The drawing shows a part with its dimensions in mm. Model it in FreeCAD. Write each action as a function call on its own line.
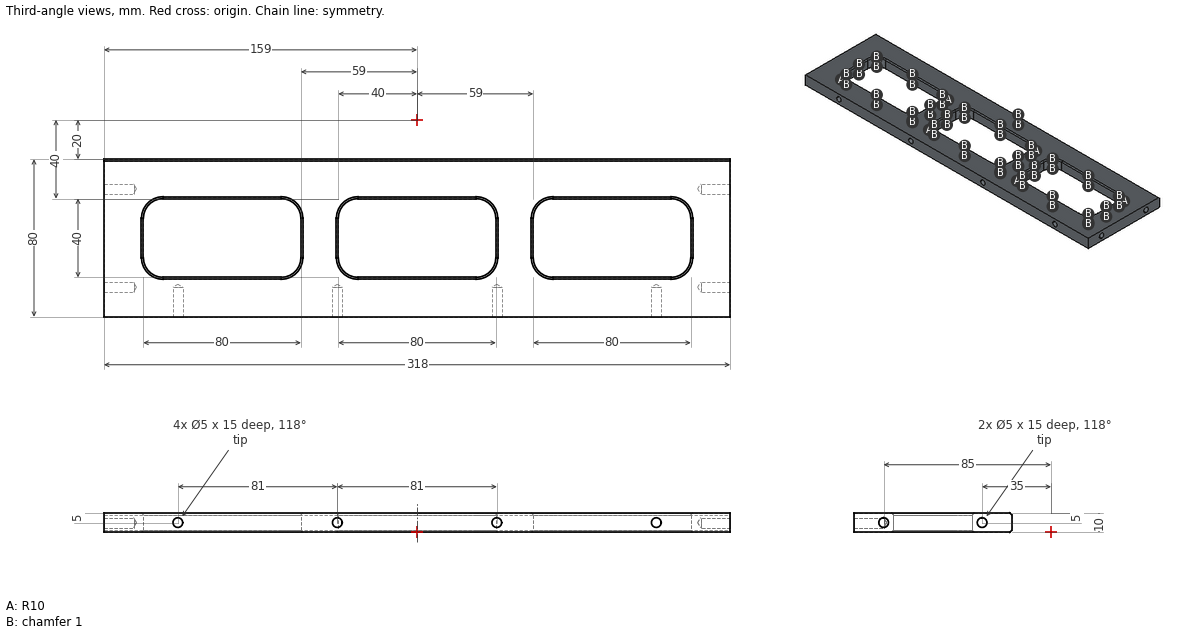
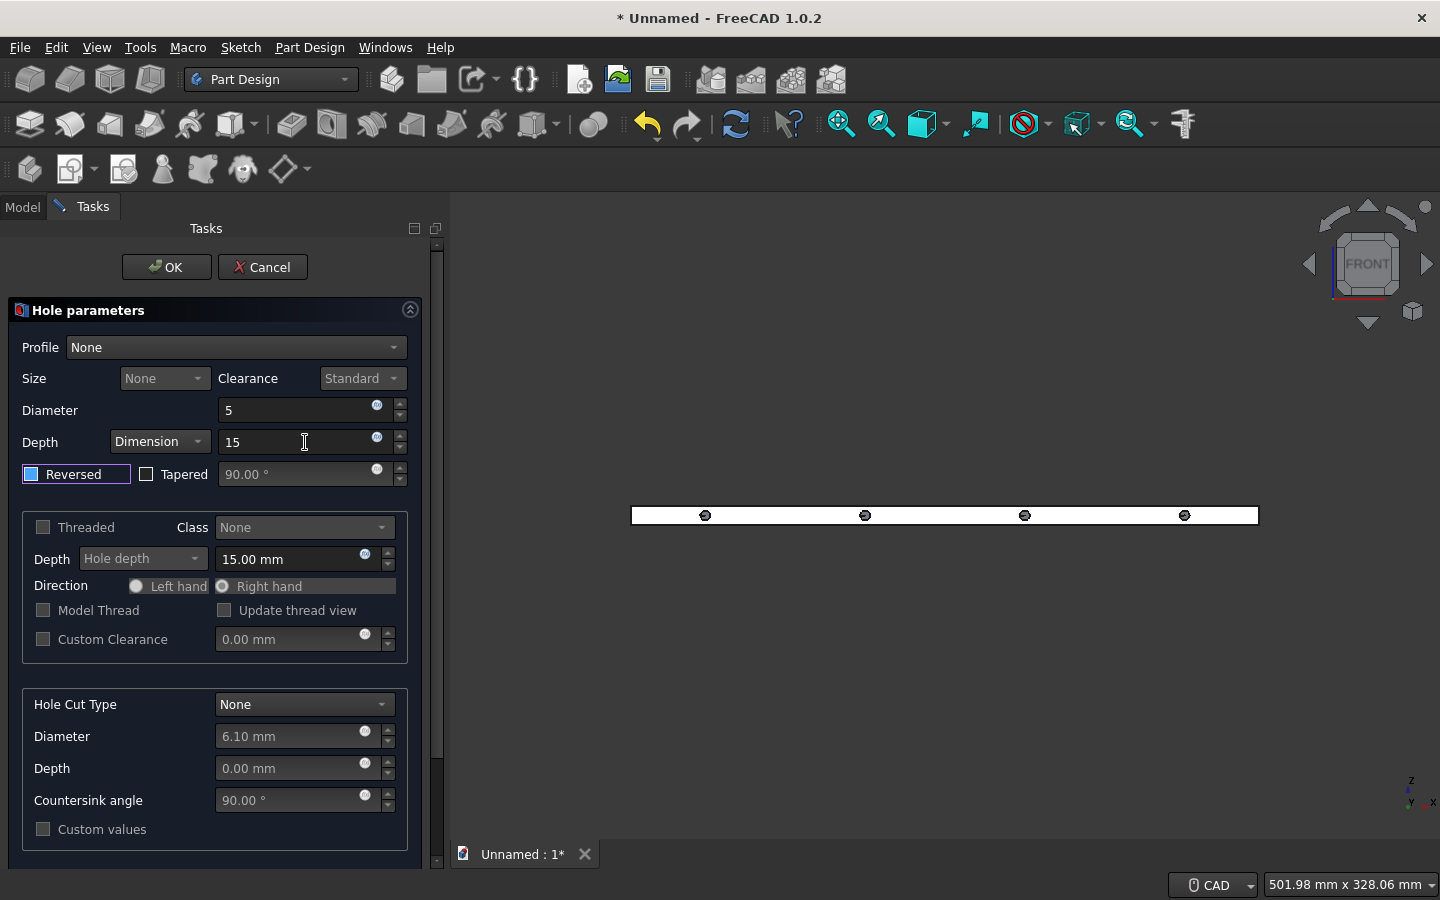
click(167, 267)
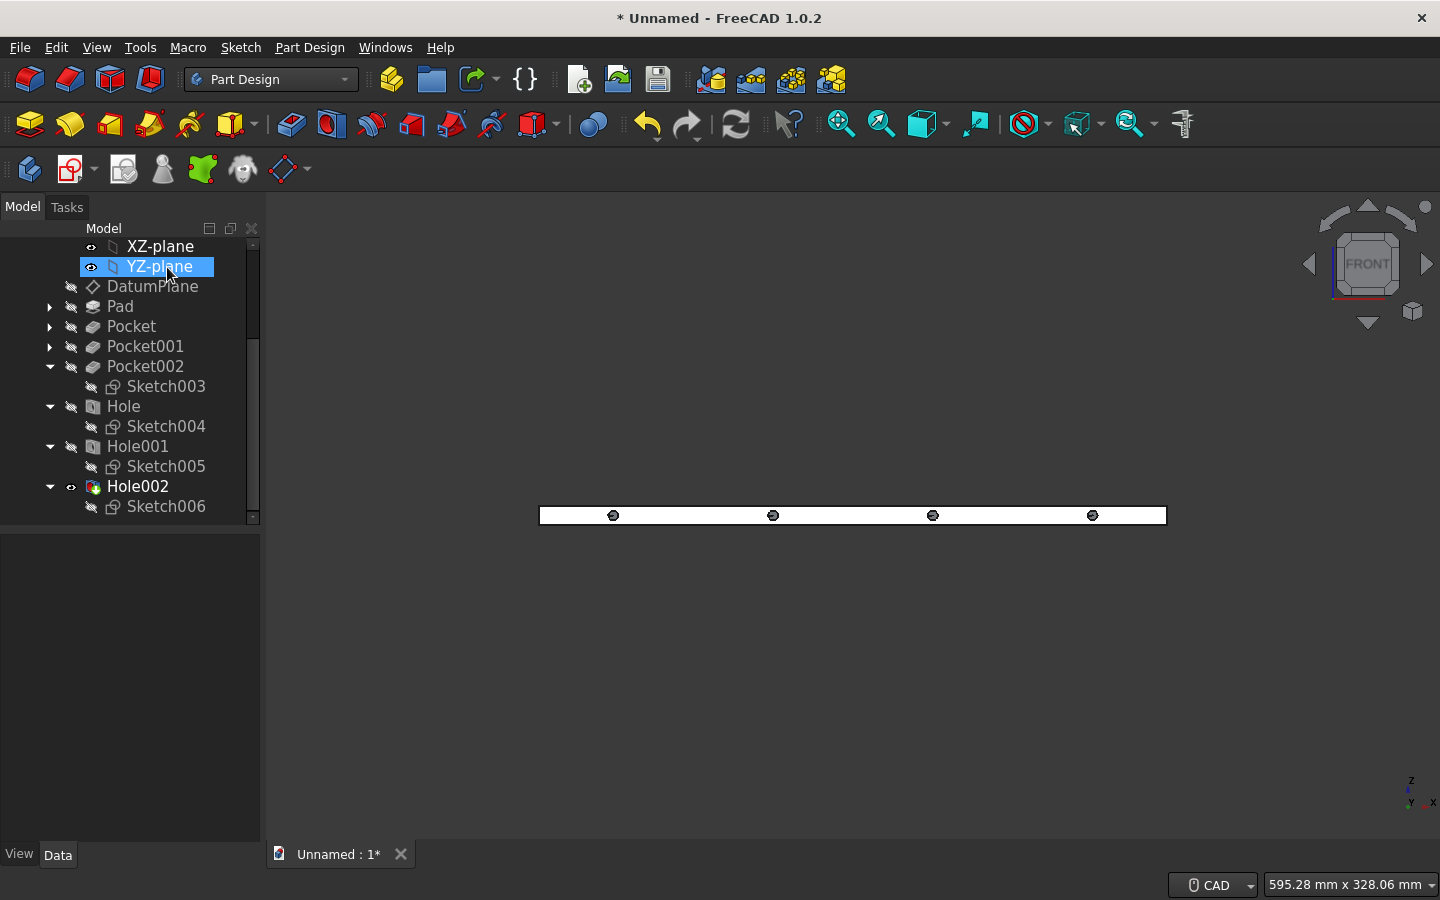
scroll(932, 514, up, 4)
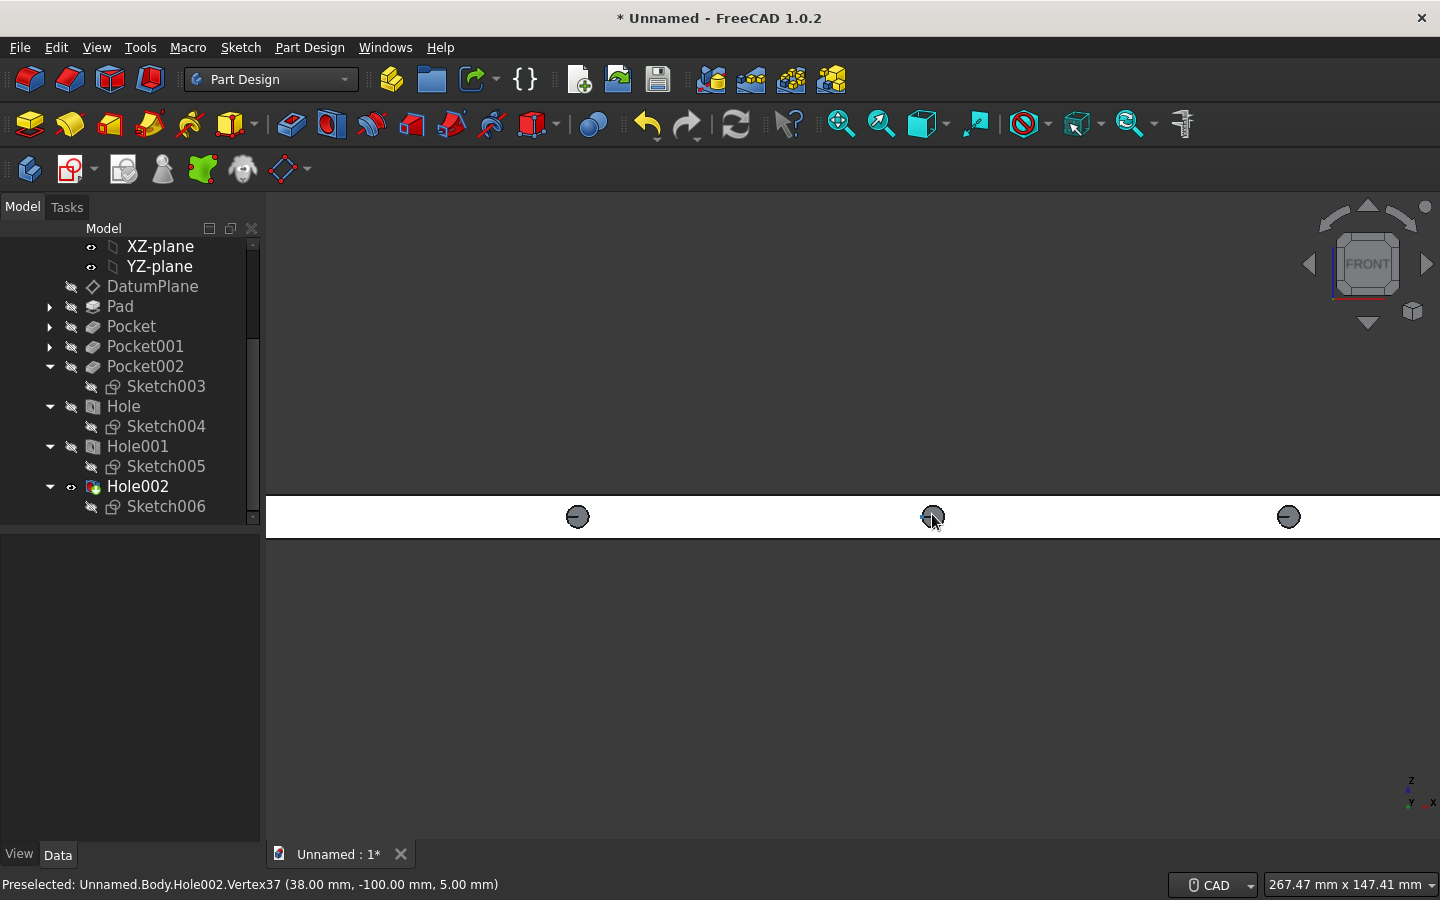
click(842, 124)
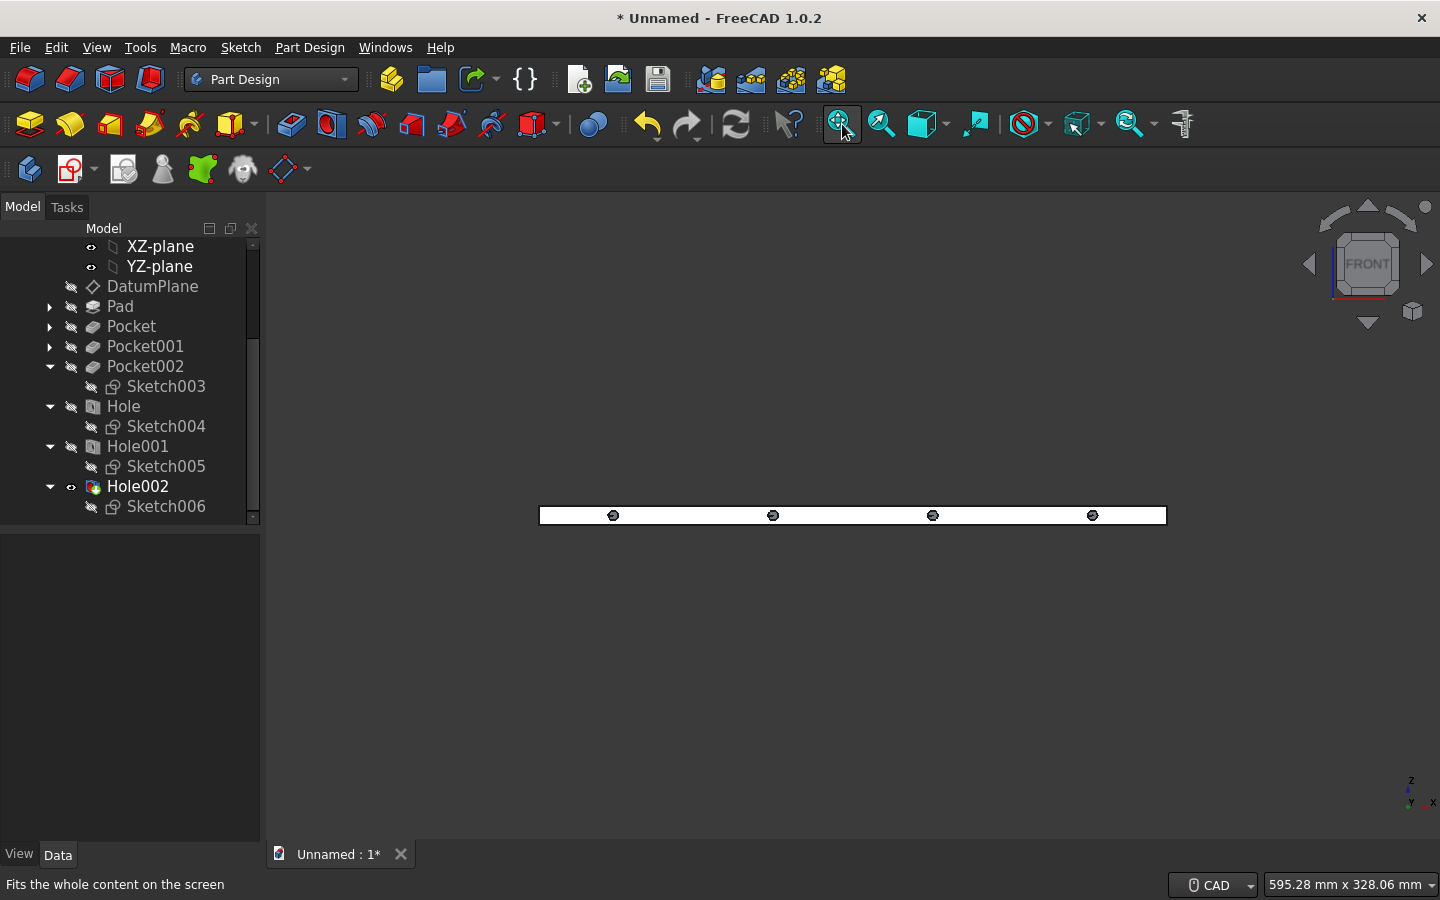
key(0)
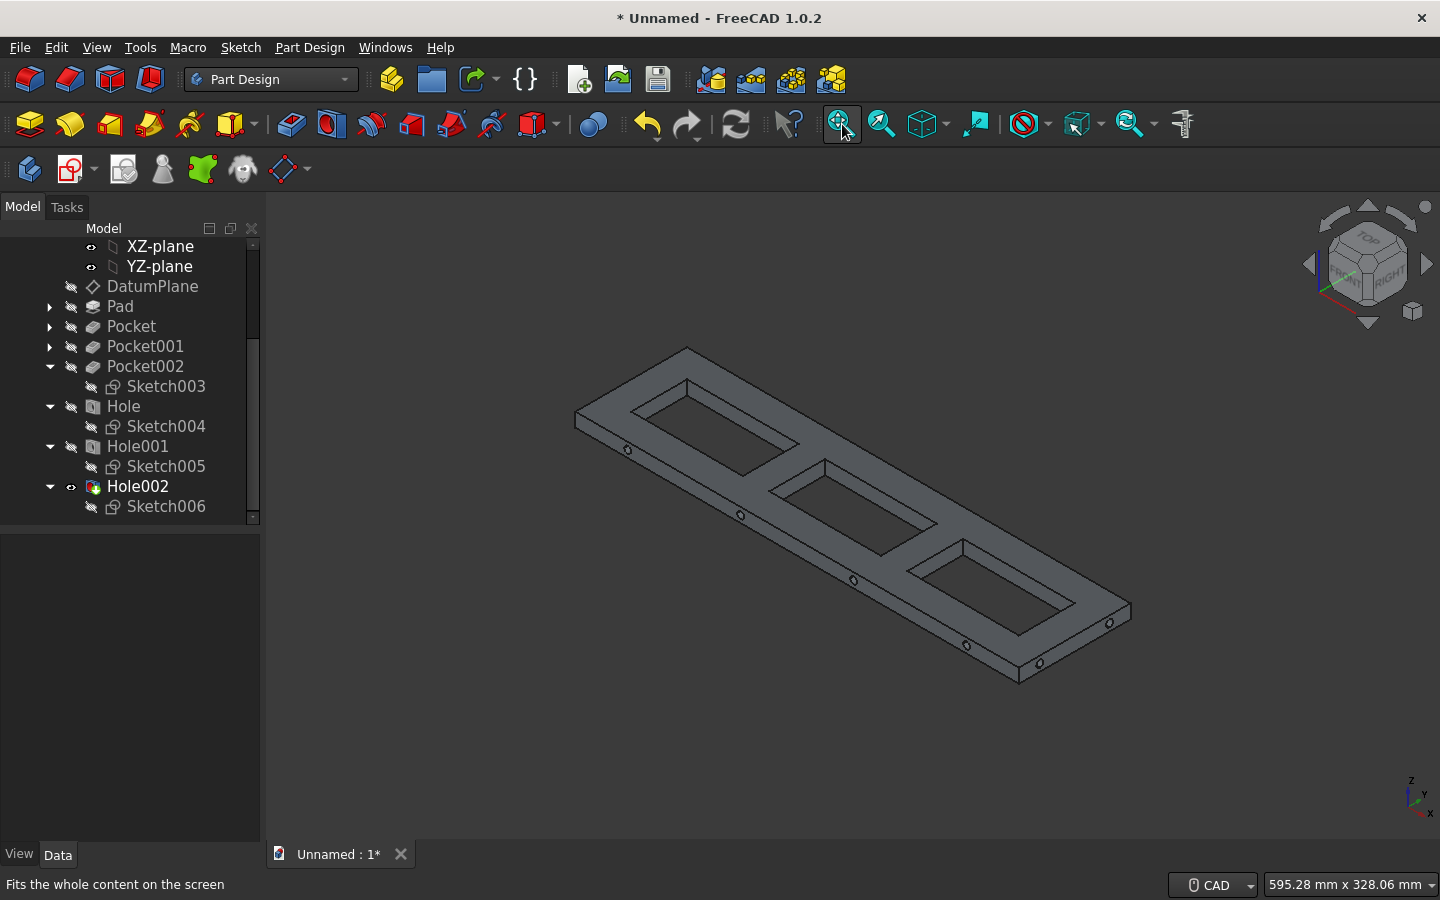
scroll(881, 563, up, 4)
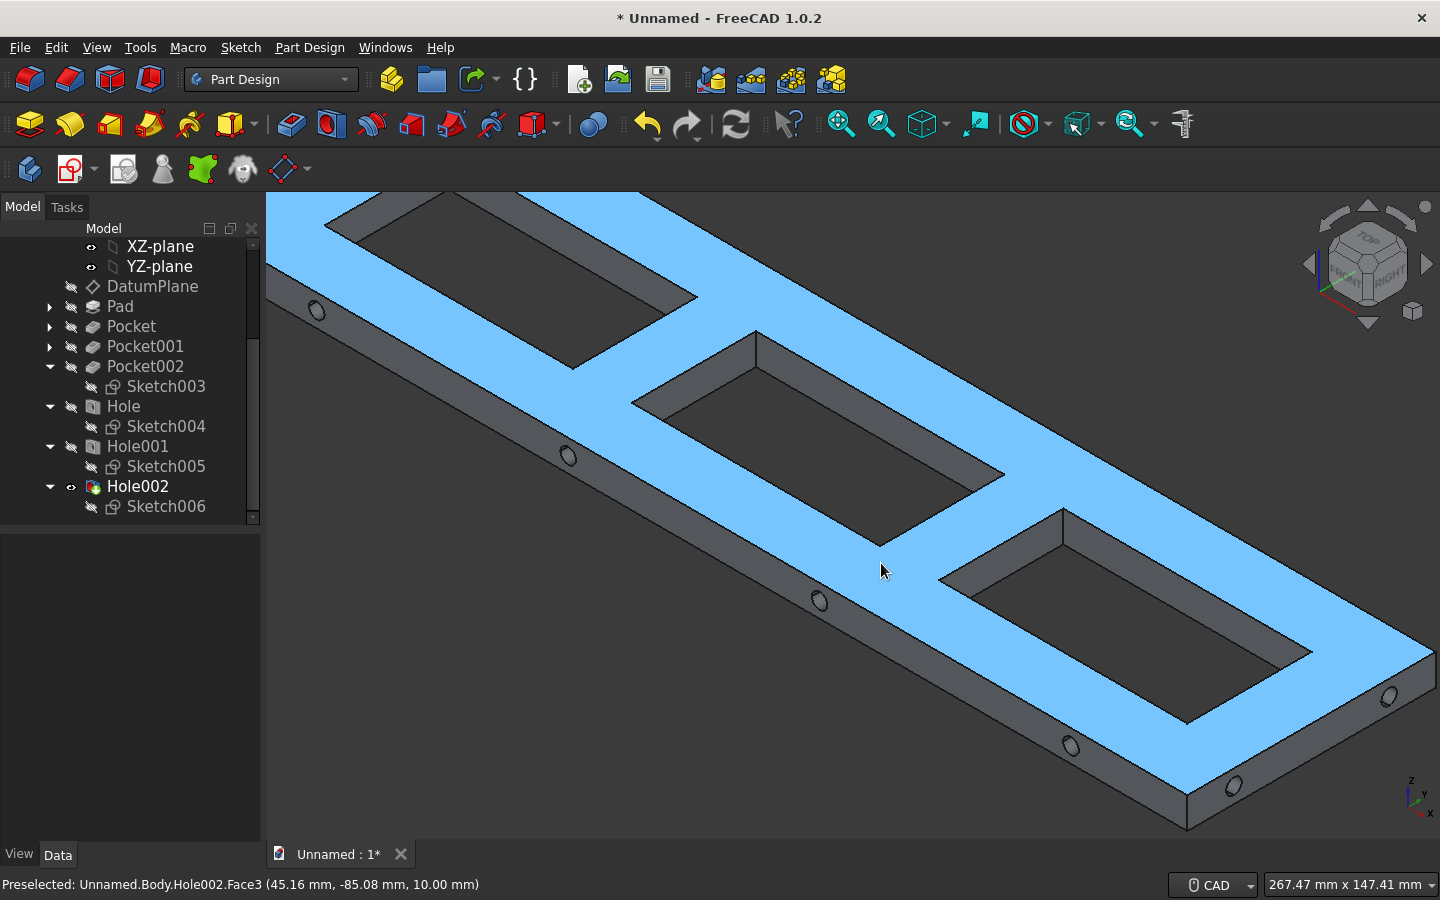
click(842, 124)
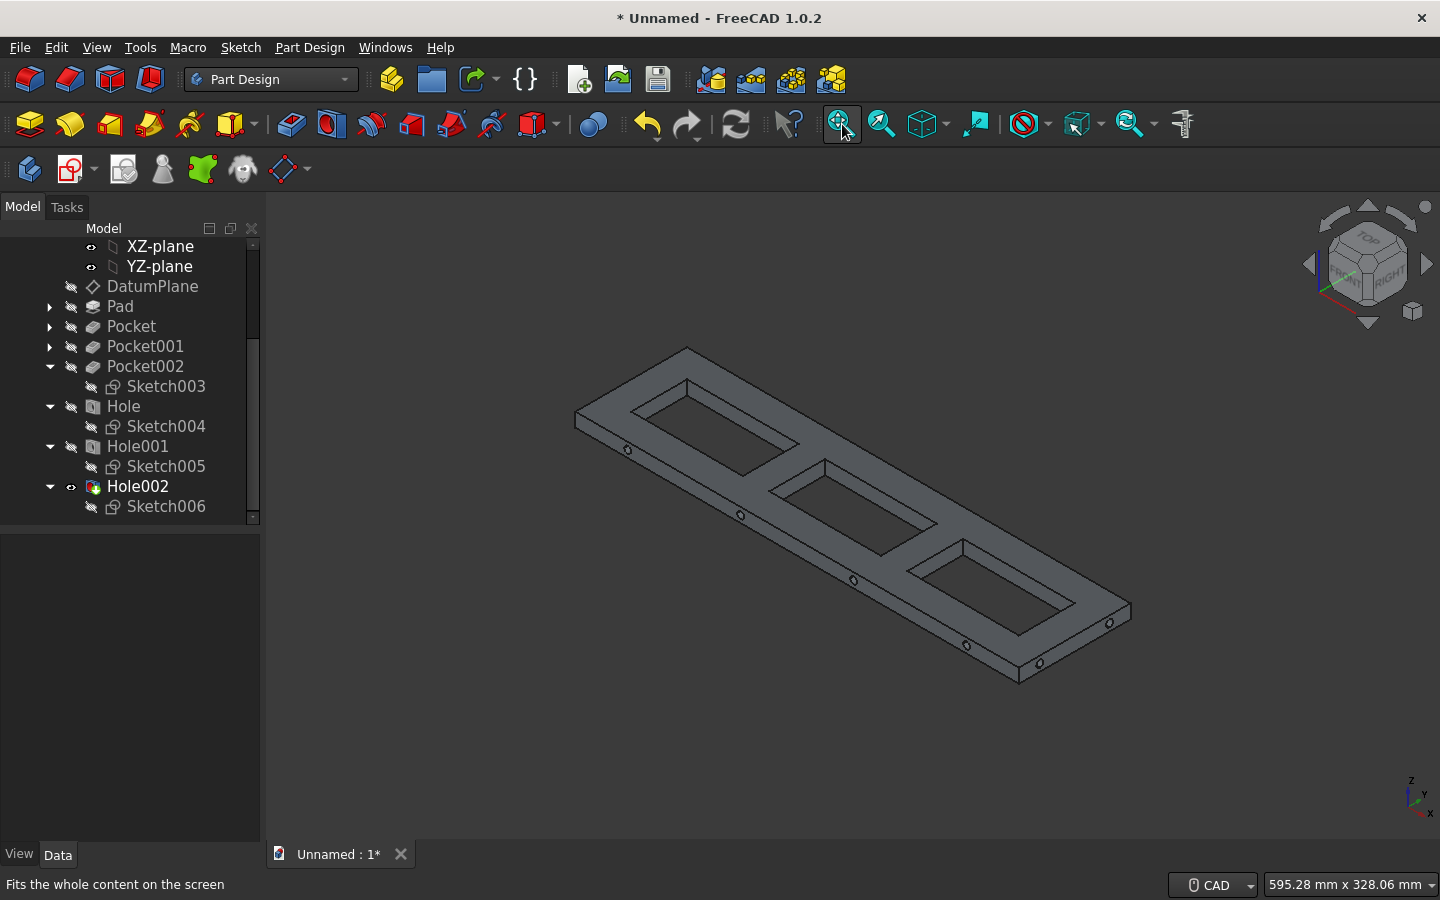
key(2)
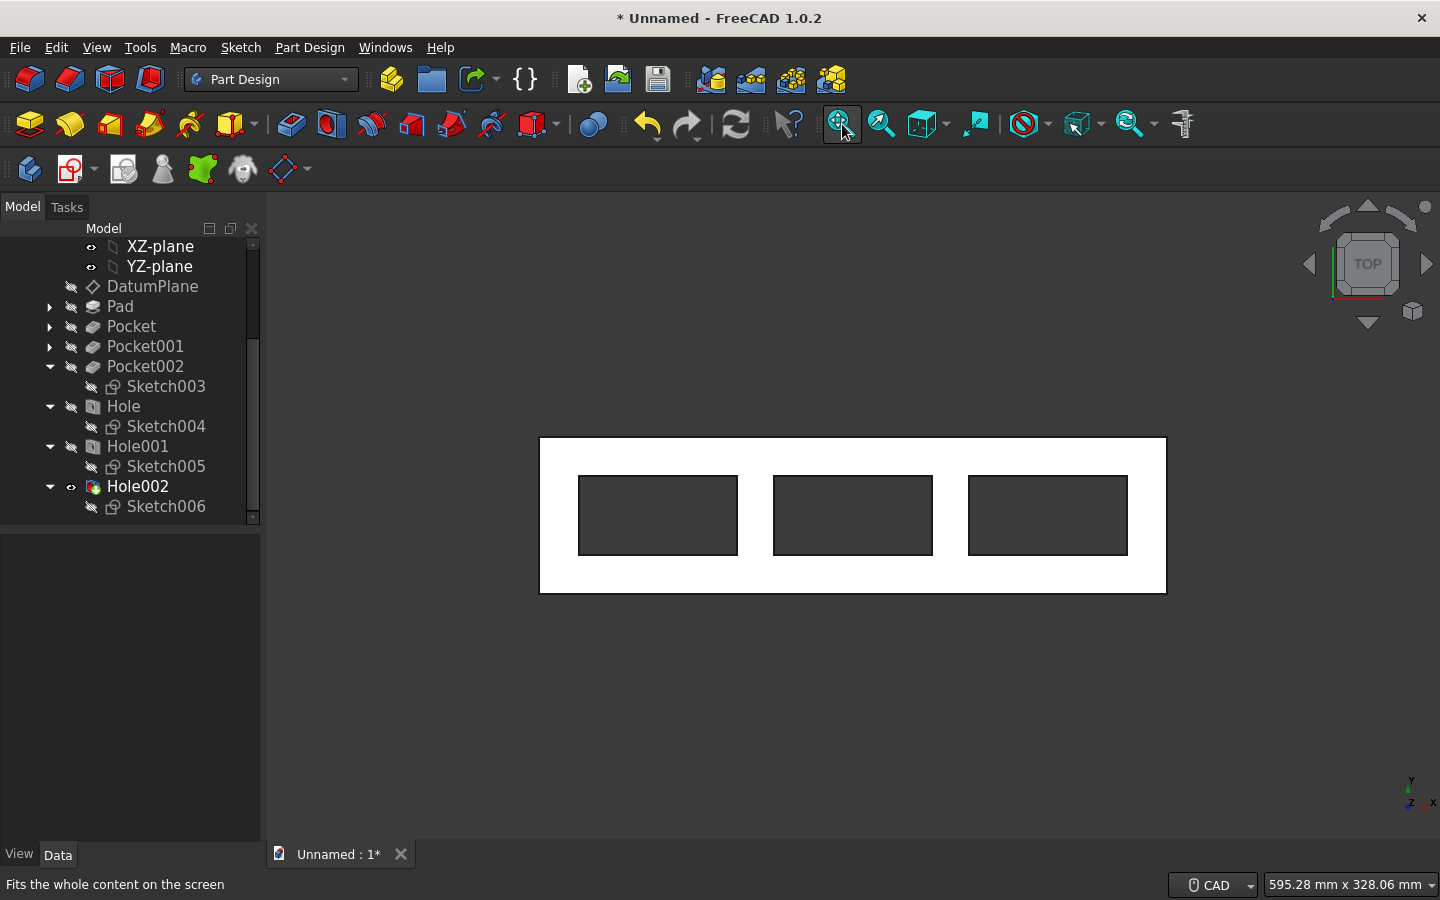
scroll(932, 554, up, 4)